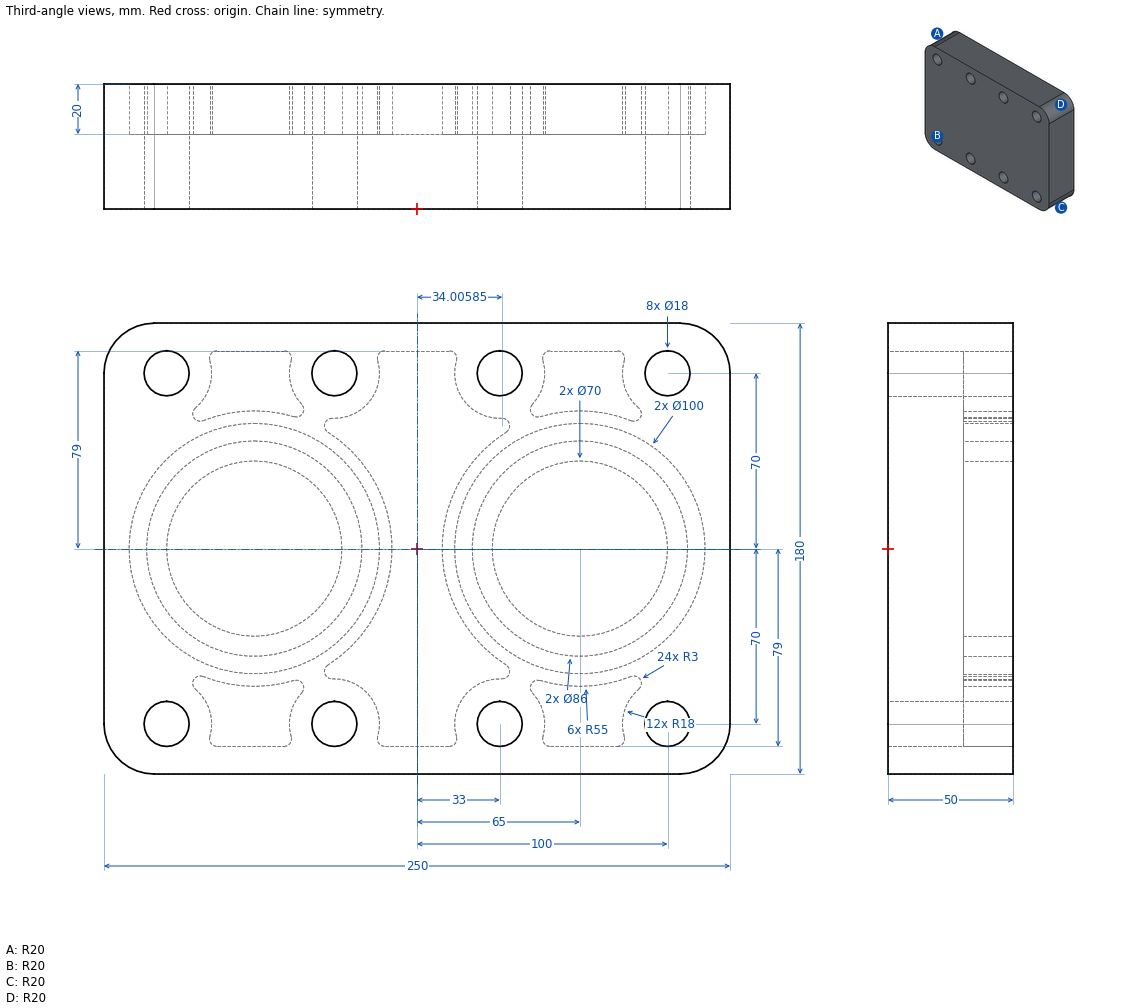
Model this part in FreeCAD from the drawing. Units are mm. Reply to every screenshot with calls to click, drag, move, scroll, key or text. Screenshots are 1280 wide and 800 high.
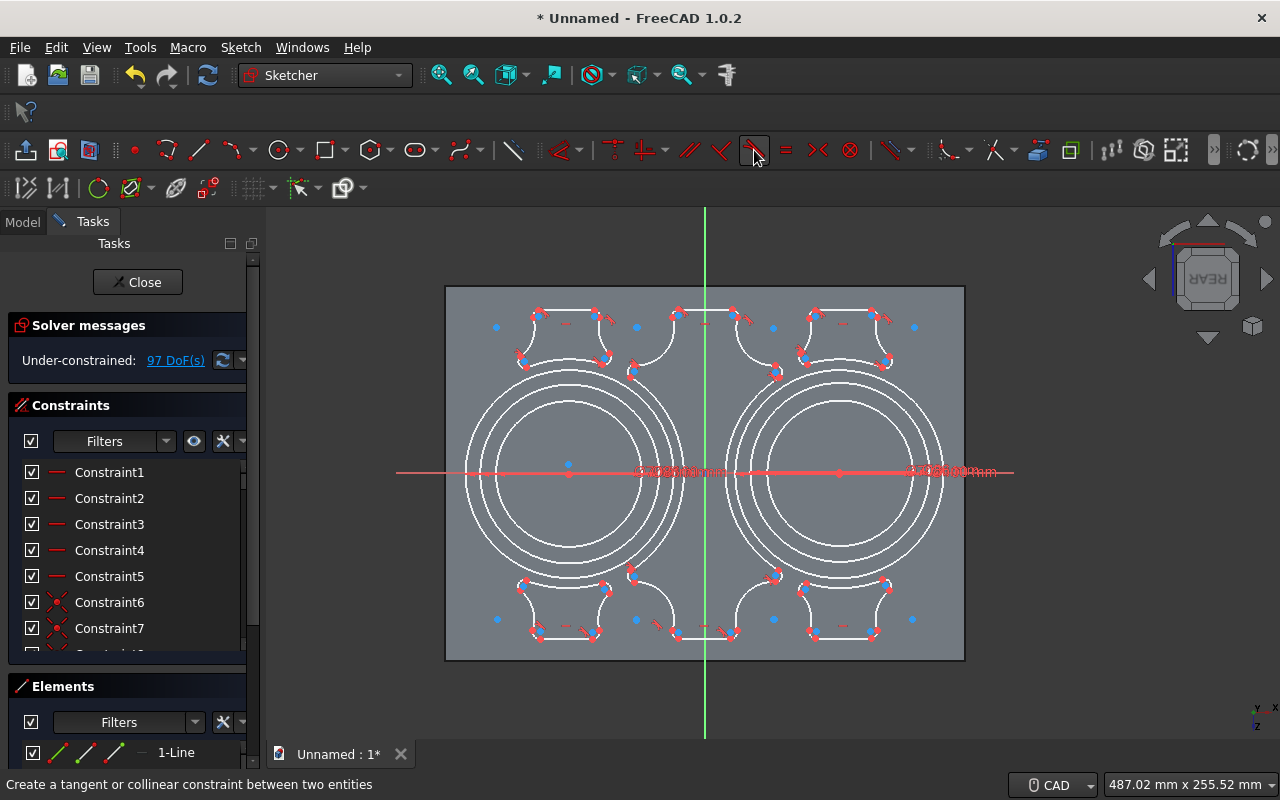
click(602, 603)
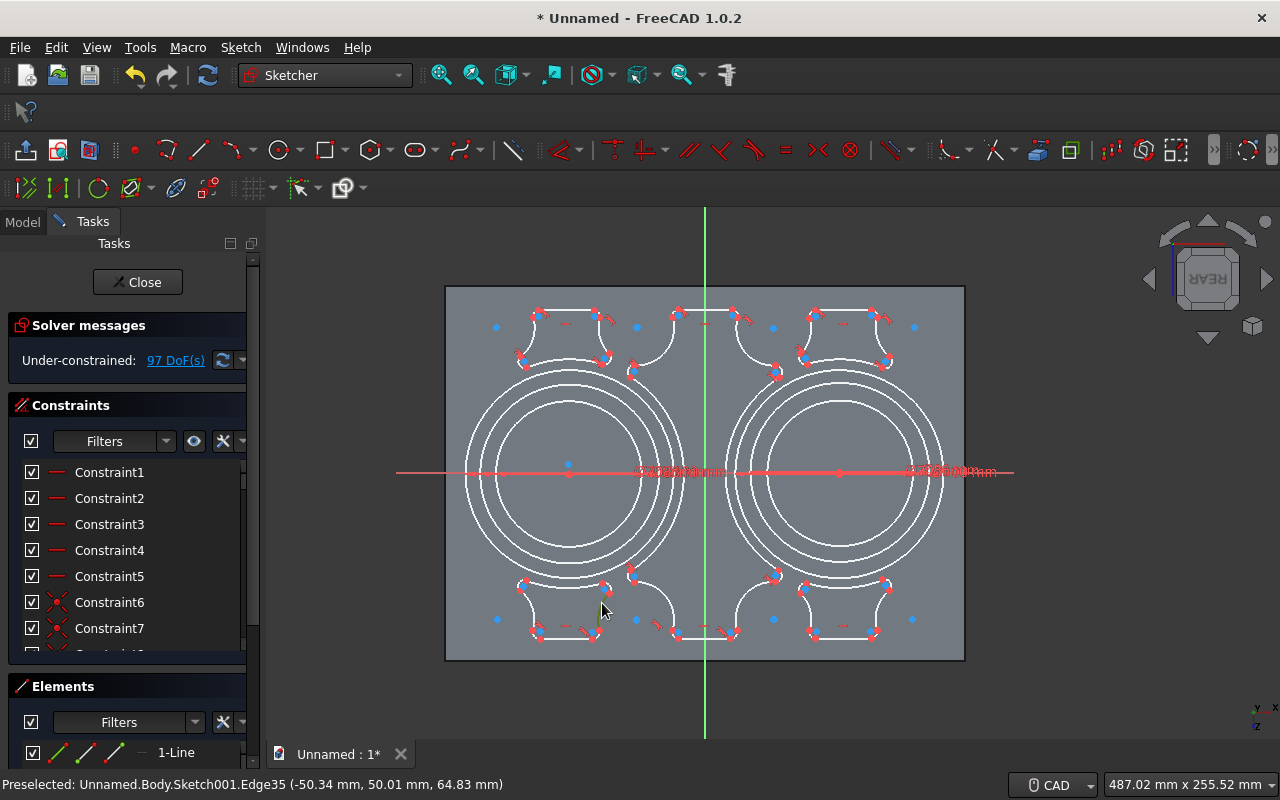
scroll(610, 586, up, 4)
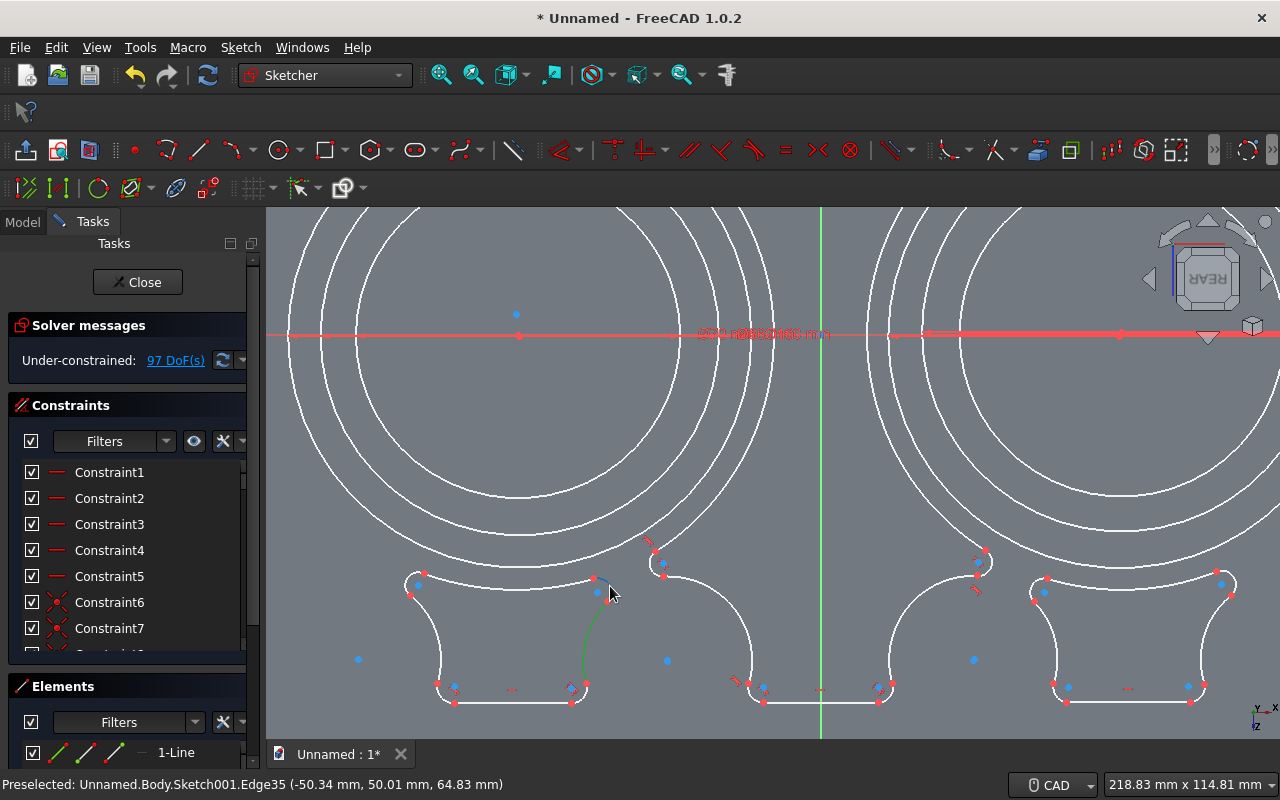
click(609, 585)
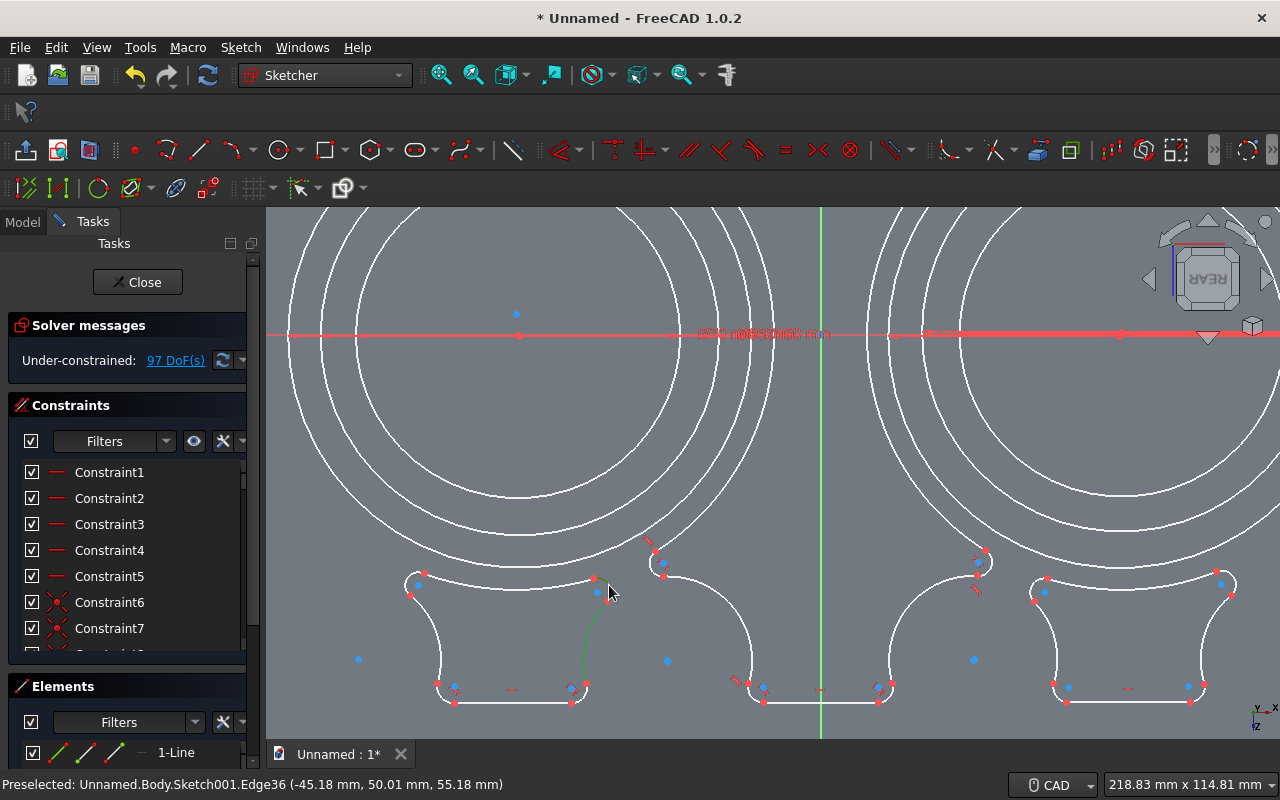
click(754, 150)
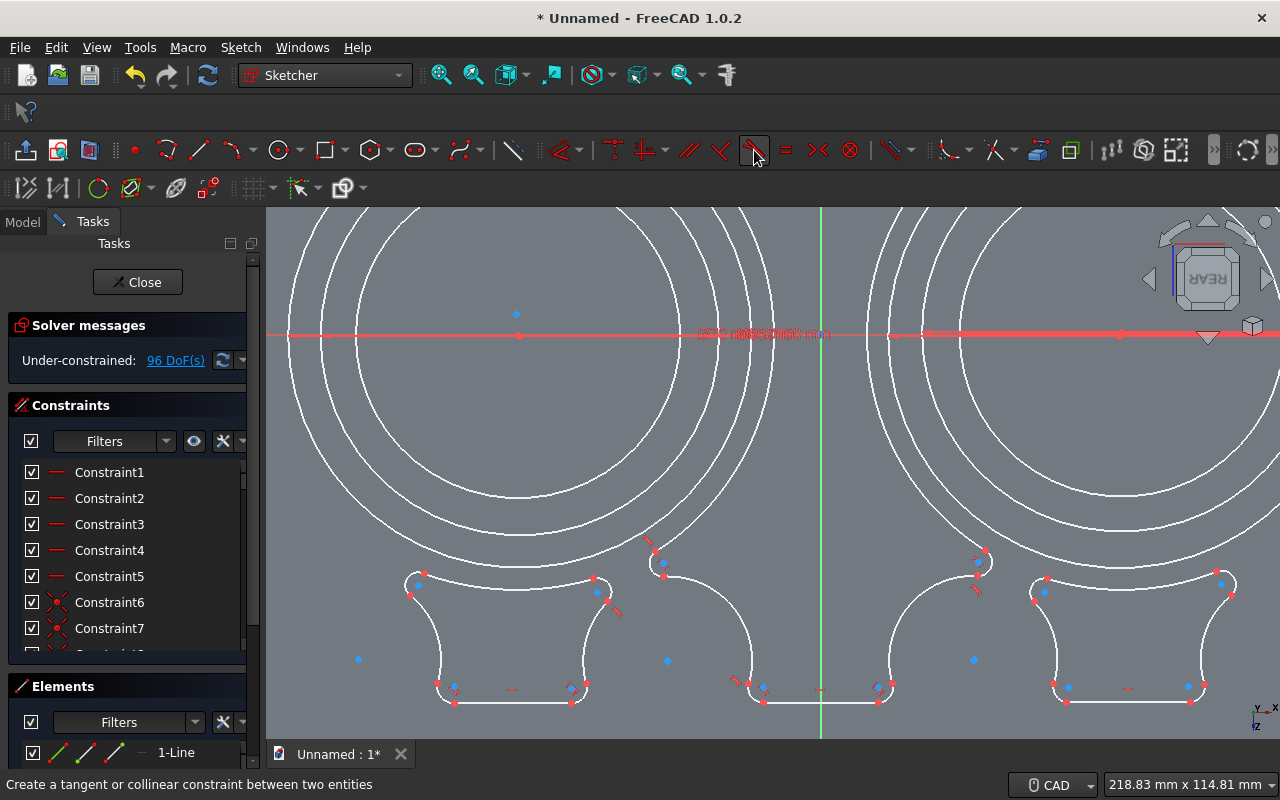
scroll(612, 592, up, 2)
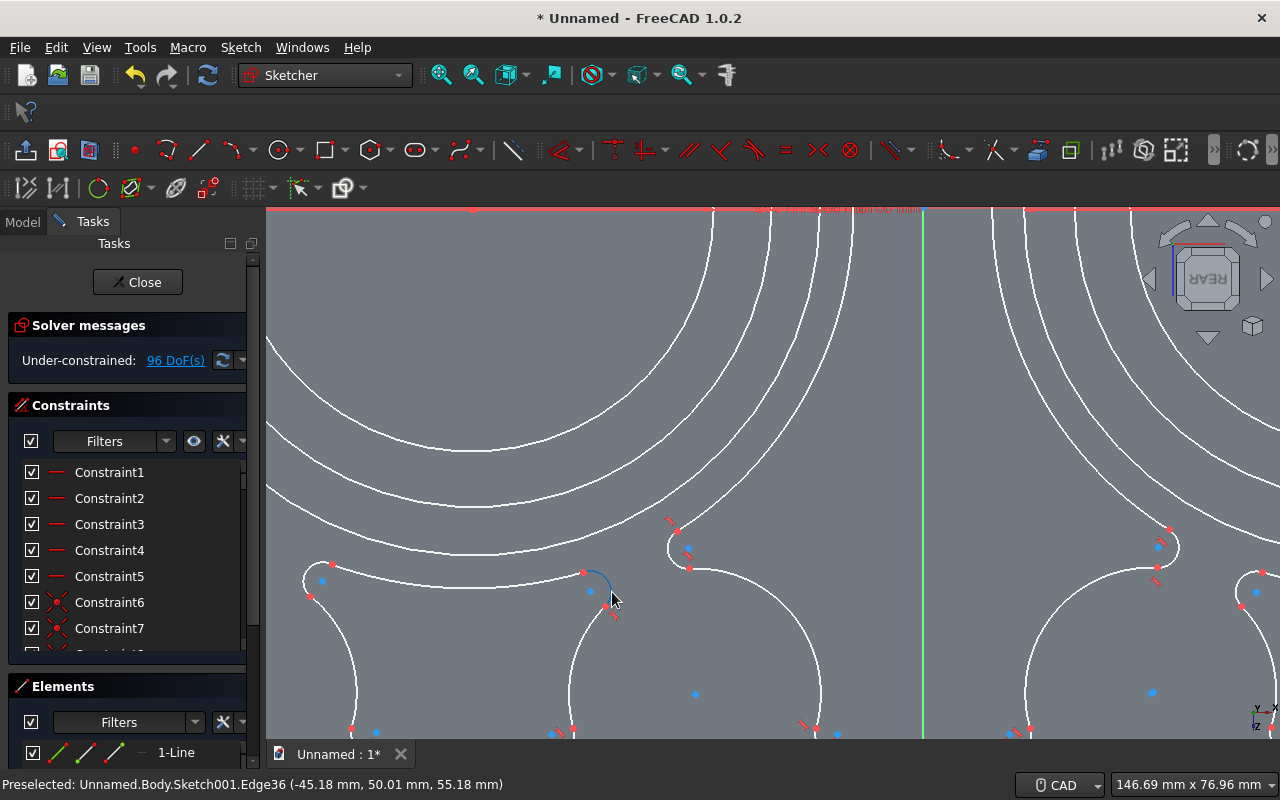
click(611, 591)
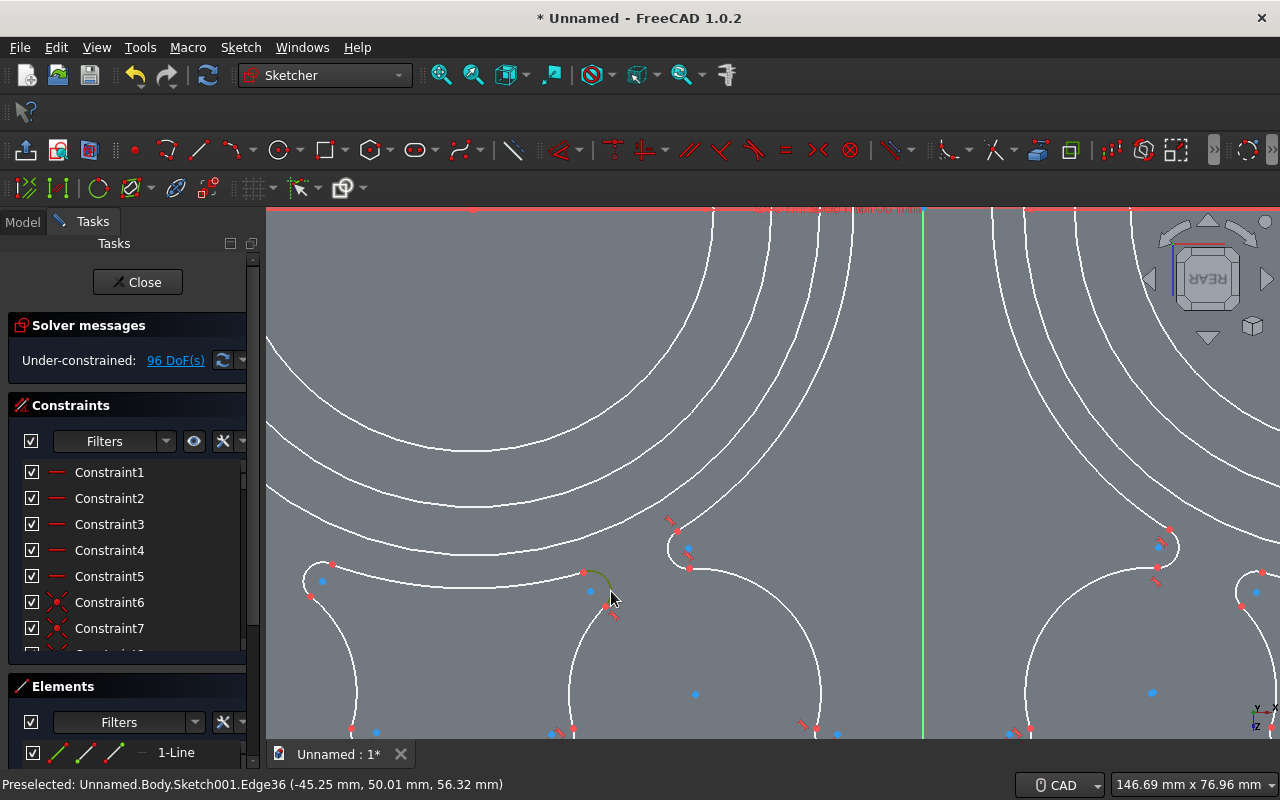
click(406, 583)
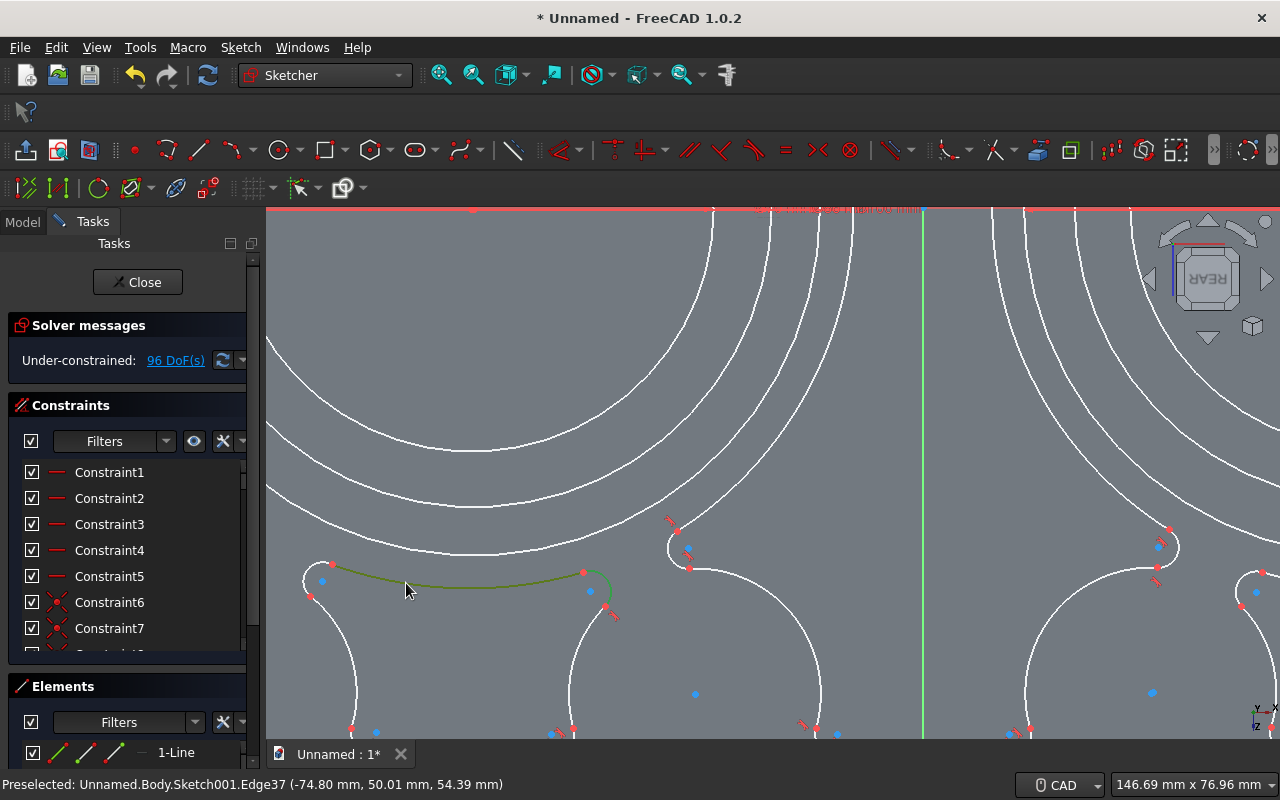
click(754, 150)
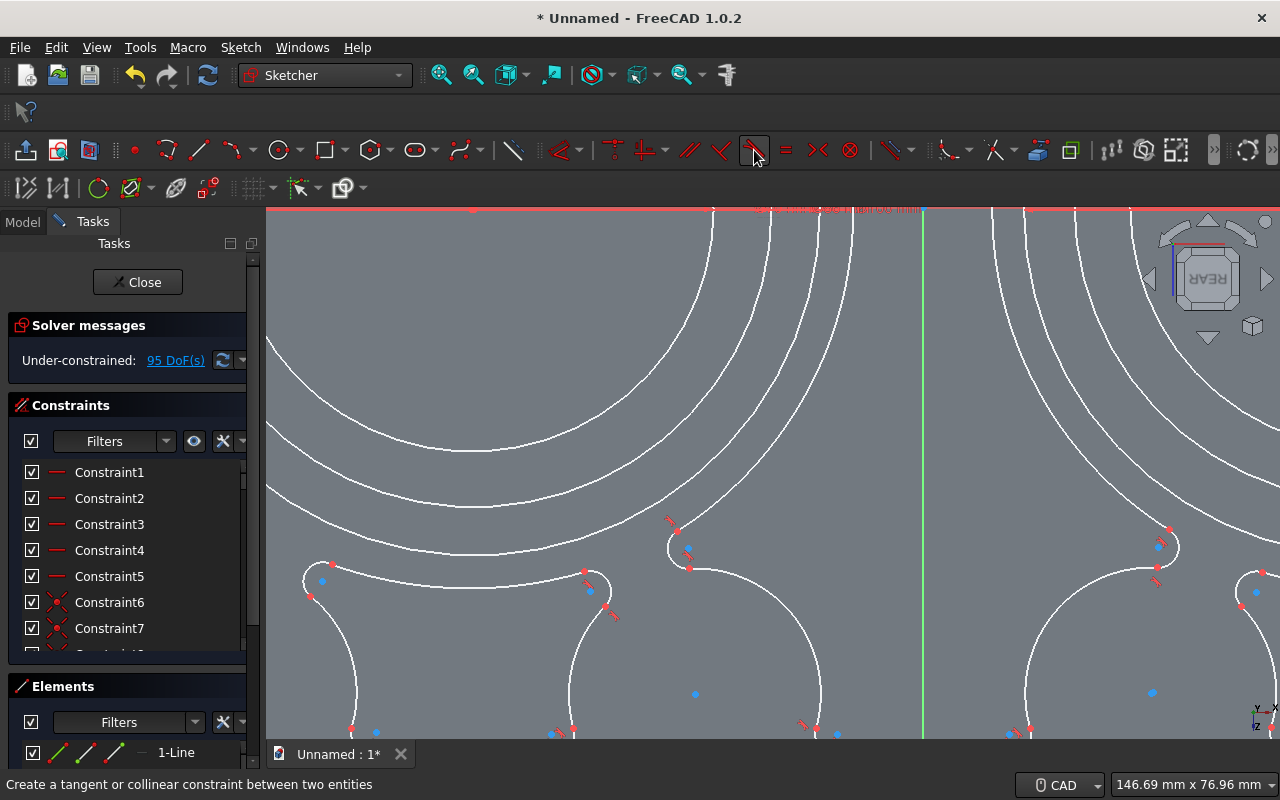
click(407, 584)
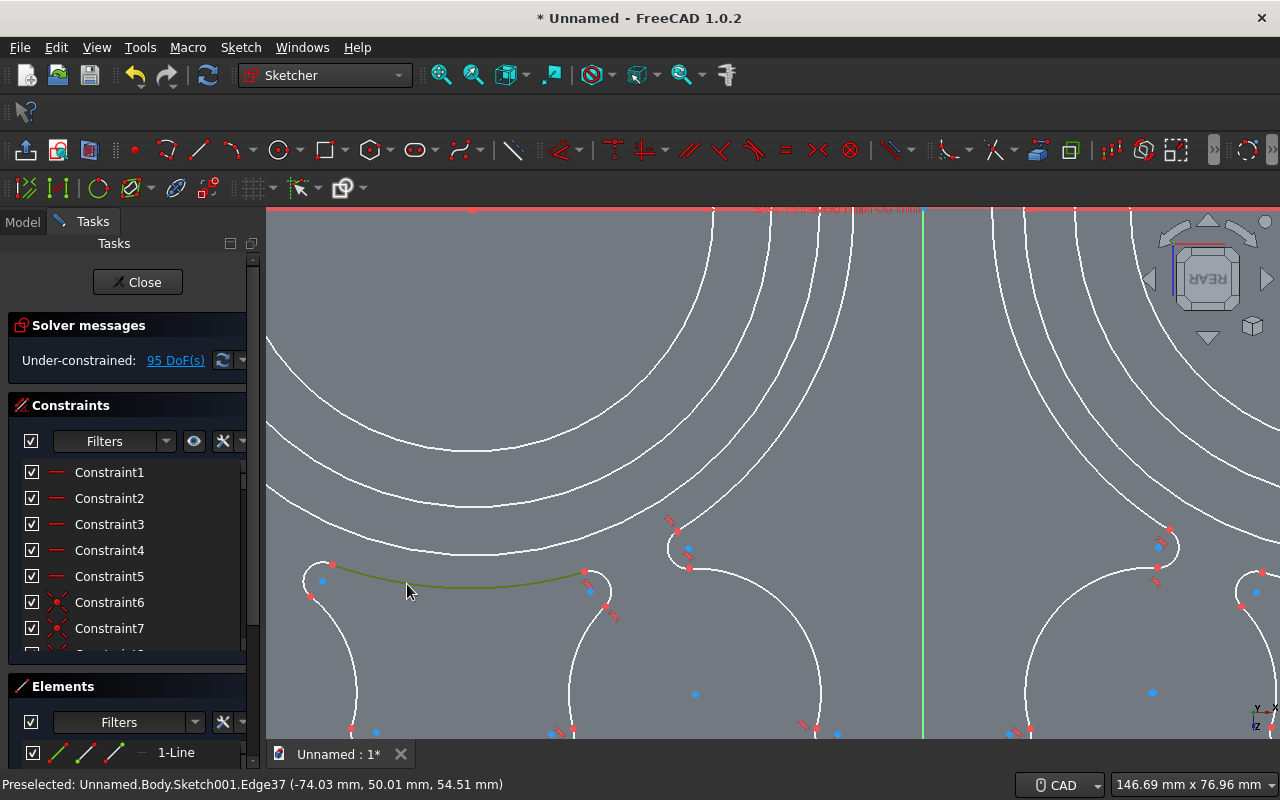
click(315, 564)